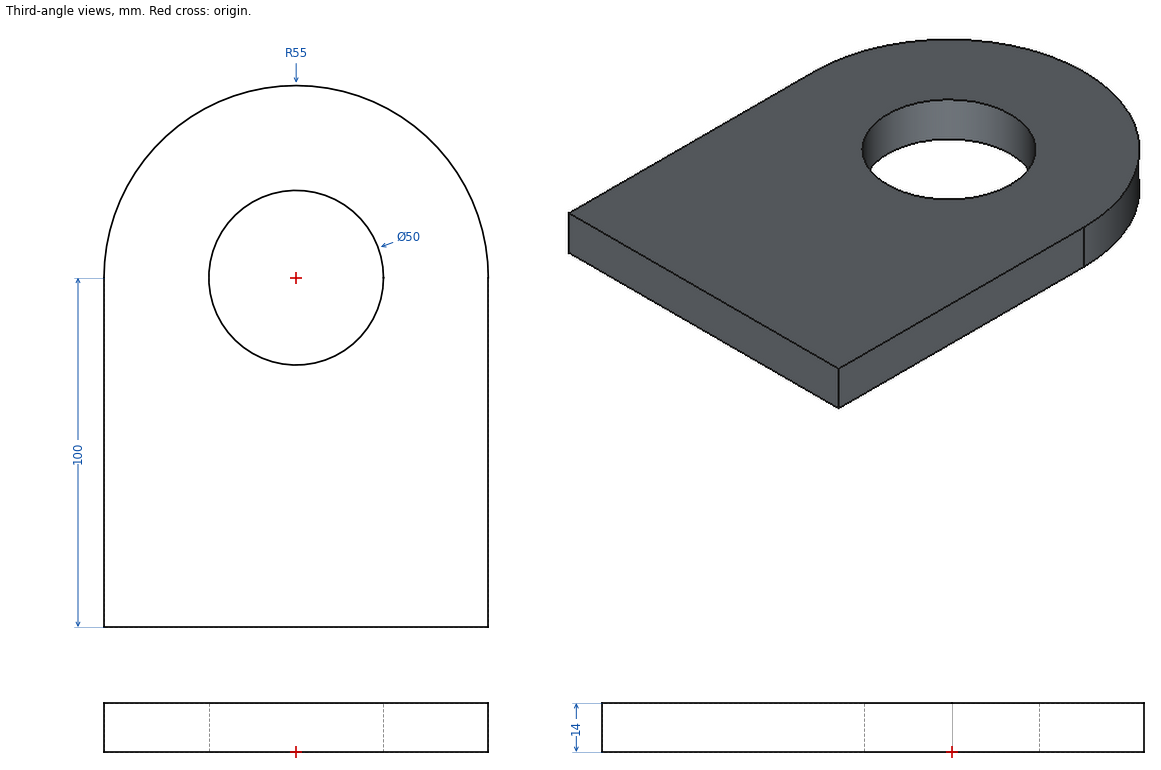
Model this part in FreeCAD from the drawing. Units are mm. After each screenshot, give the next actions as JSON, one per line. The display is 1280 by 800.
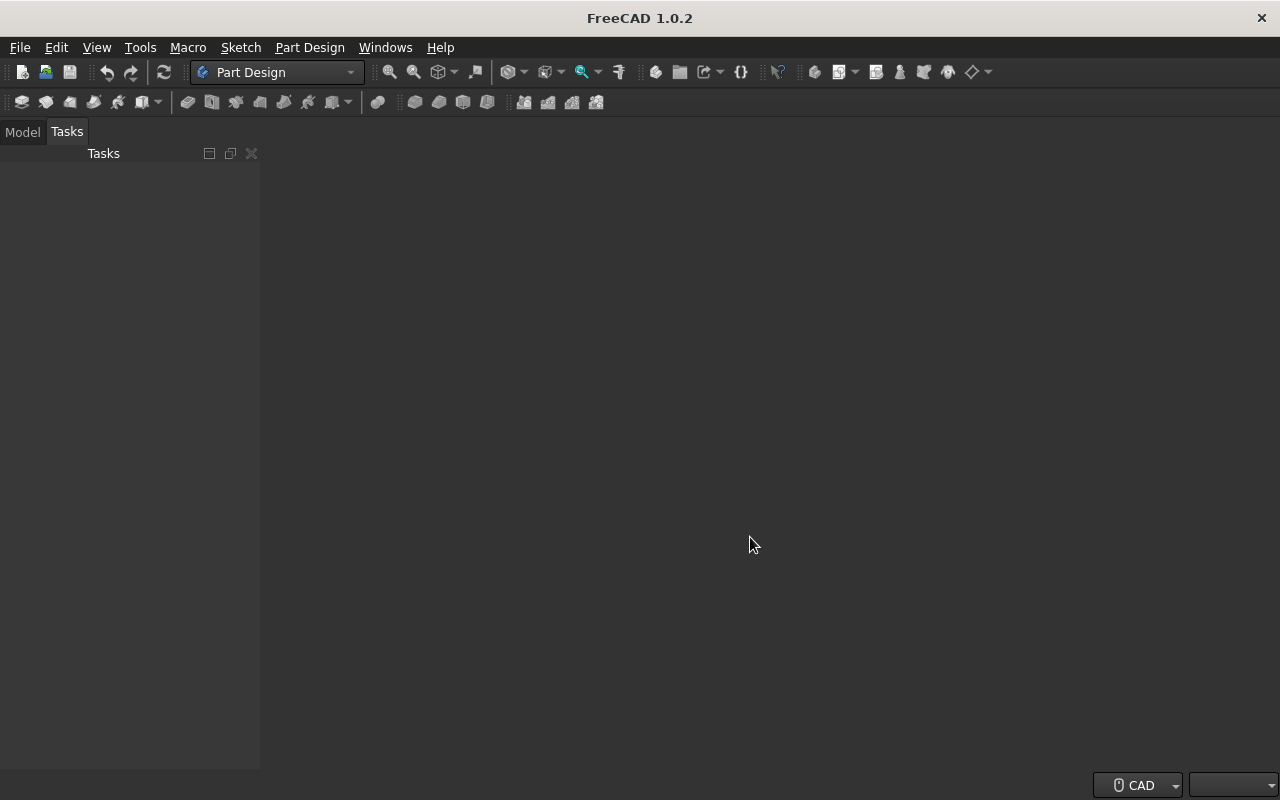
{"action": "left_click", "coordinate": [22, 72]}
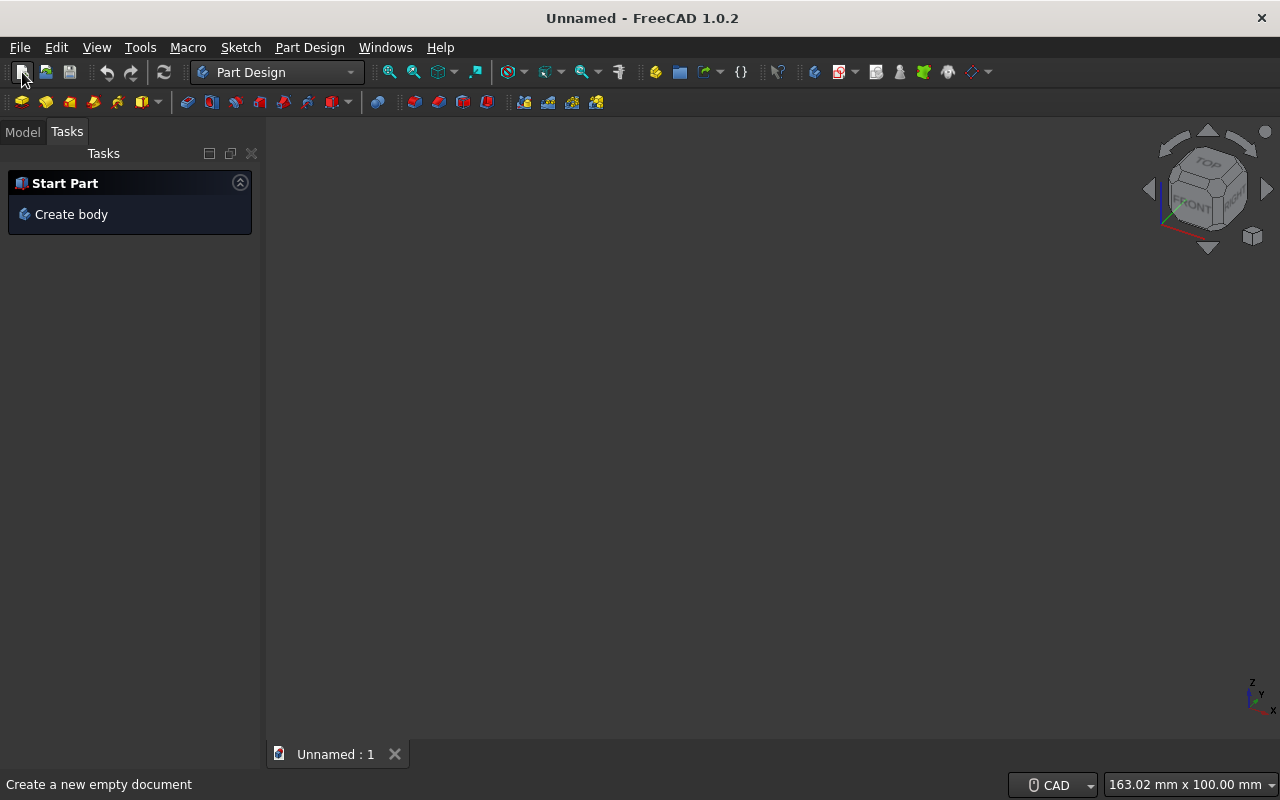
{"action": "left_click", "coordinate": [840, 72]}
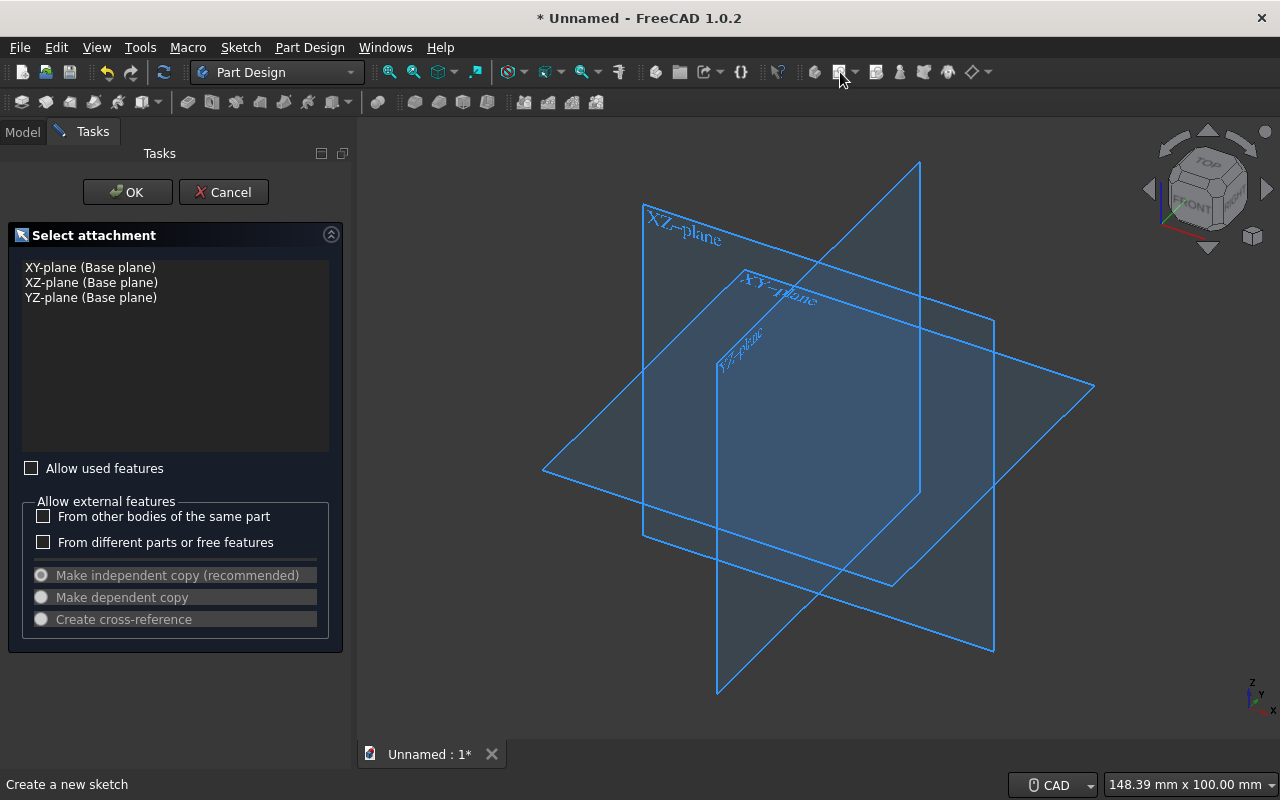
{"action": "left_click", "coordinate": [82, 268]}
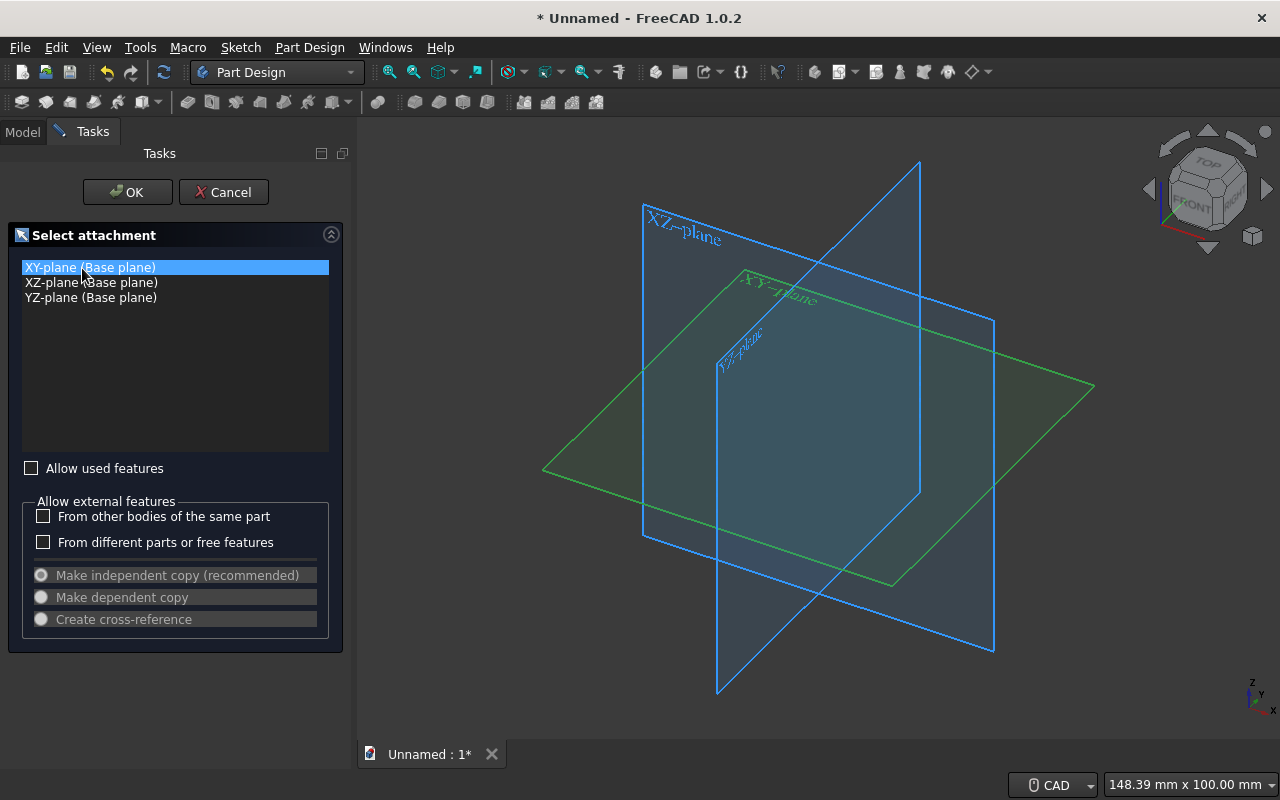
{"action": "left_click", "coordinate": [128, 192]}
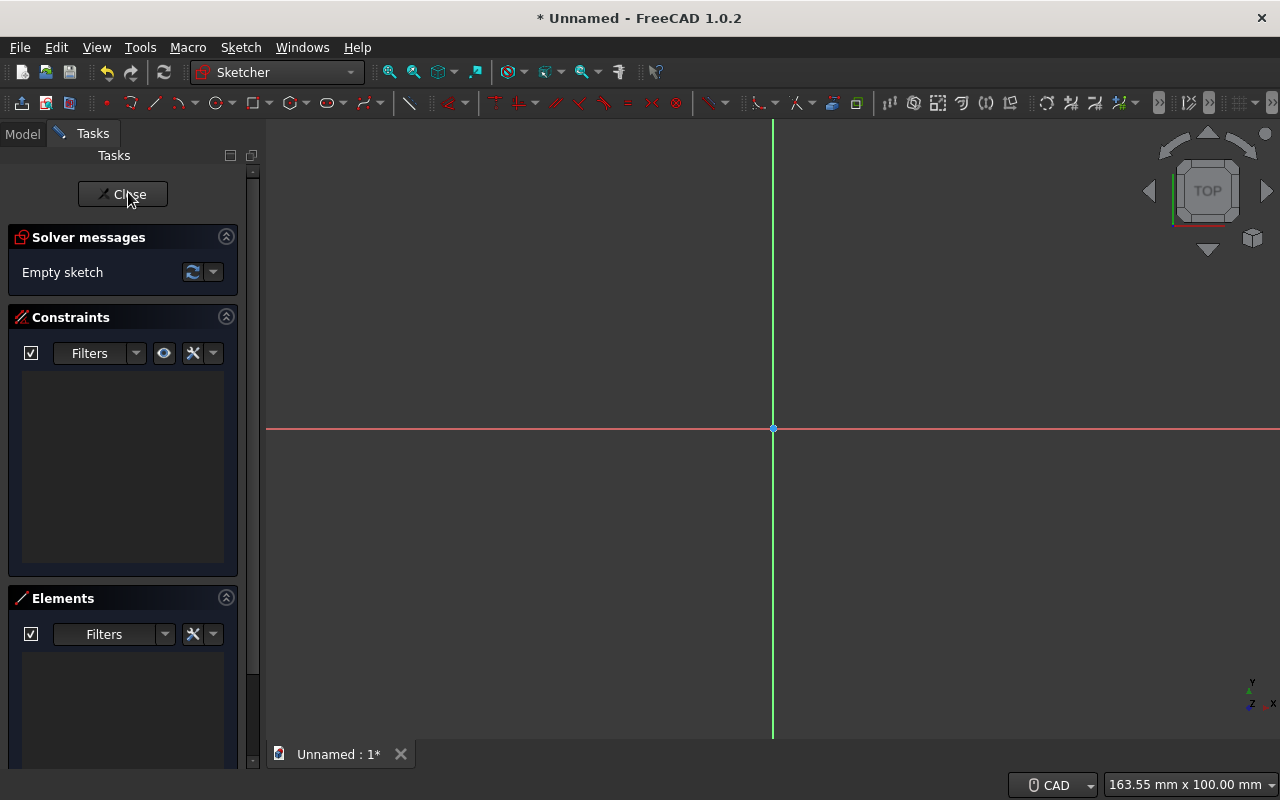
{"action": "scroll", "coordinate": [649, 315], "scroll_direction": "down", "scroll_amount": 4}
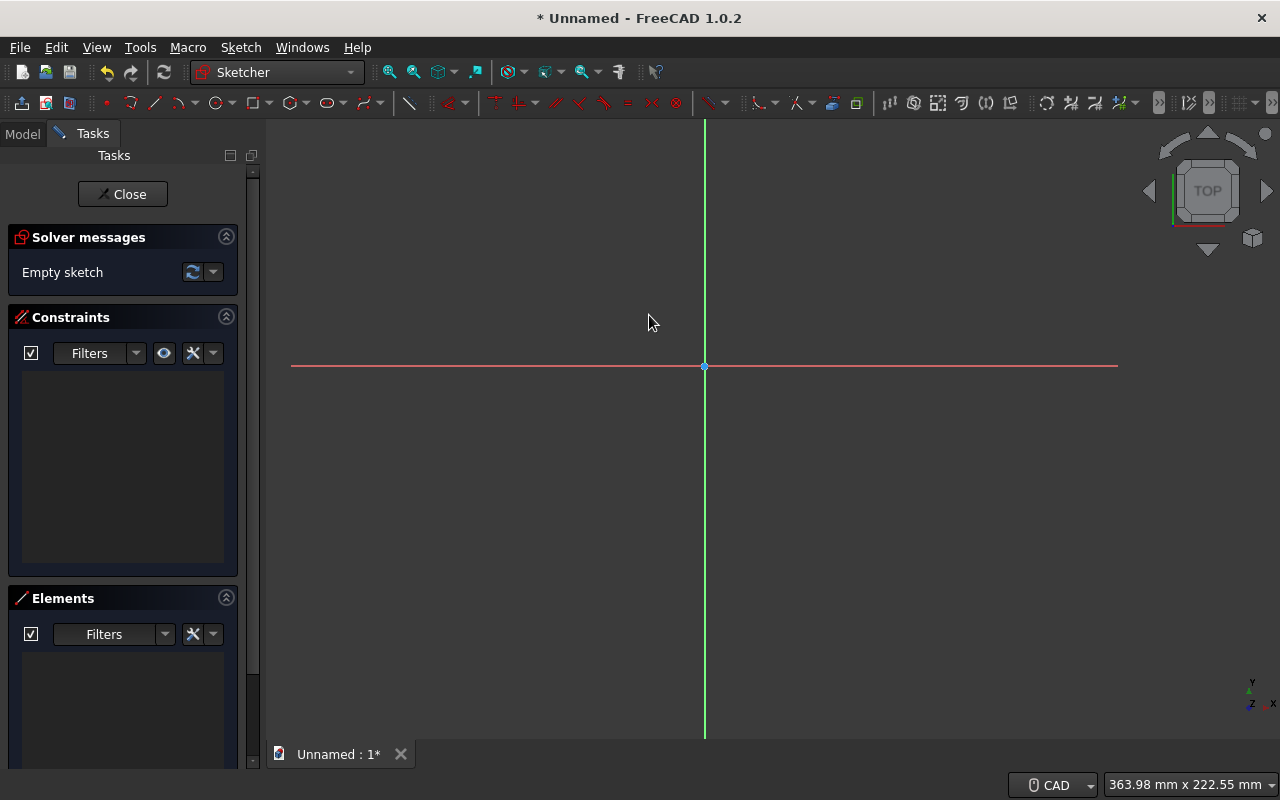
{"action": "key", "text": "g m"}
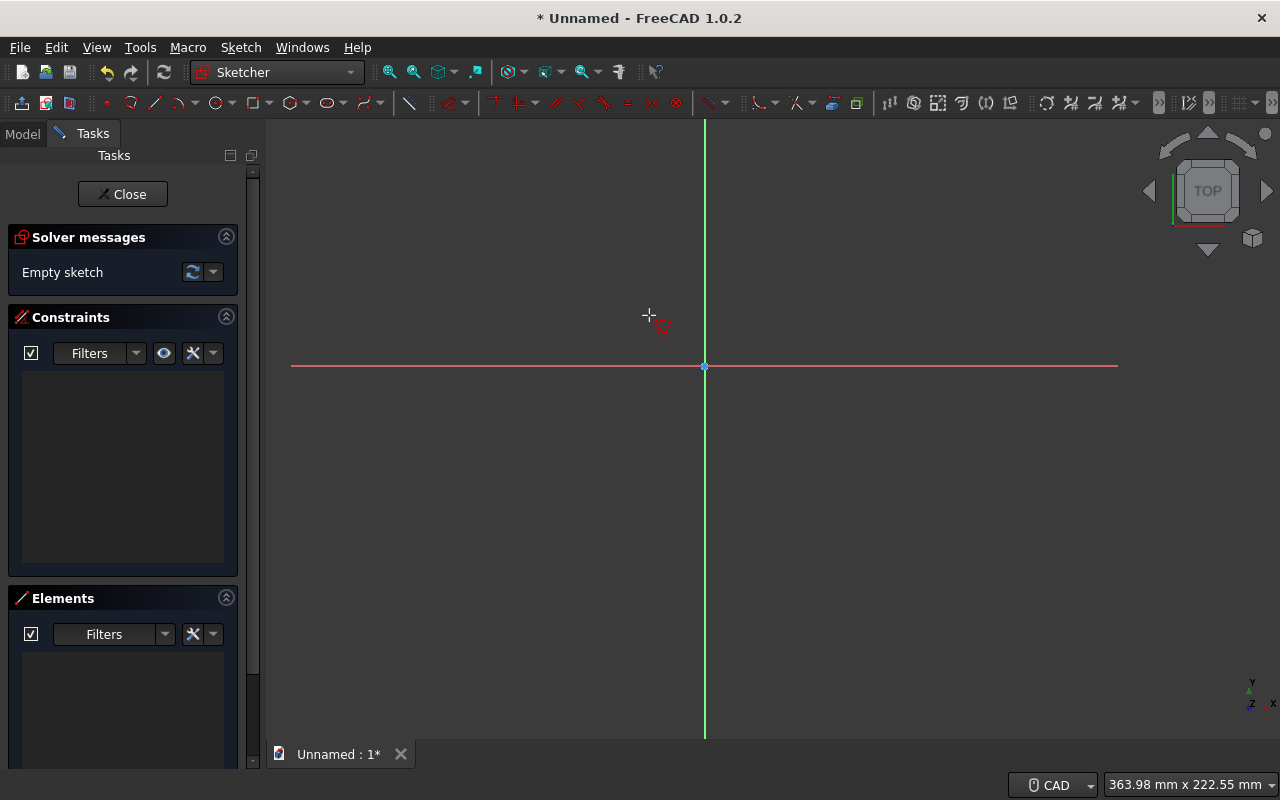
{"action": "left_click", "coordinate": [552, 366]}
{"action": "left_click", "coordinate": [552, 645]}
{"action": "left_click", "coordinate": [858, 645]}
{"action": "left_click", "coordinate": [858, 366]}
{"action": "right_click", "coordinate": [858, 366]}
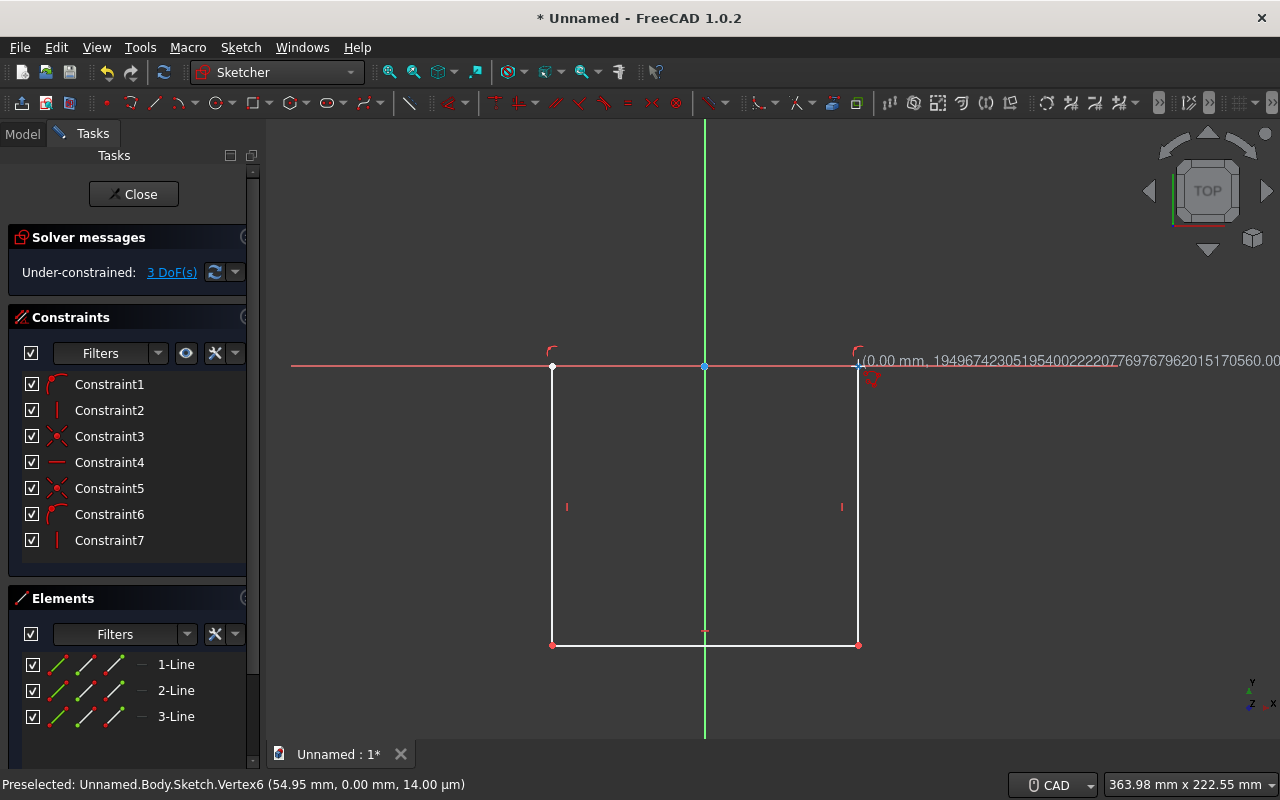
{"action": "key", "text": "g 3 a"}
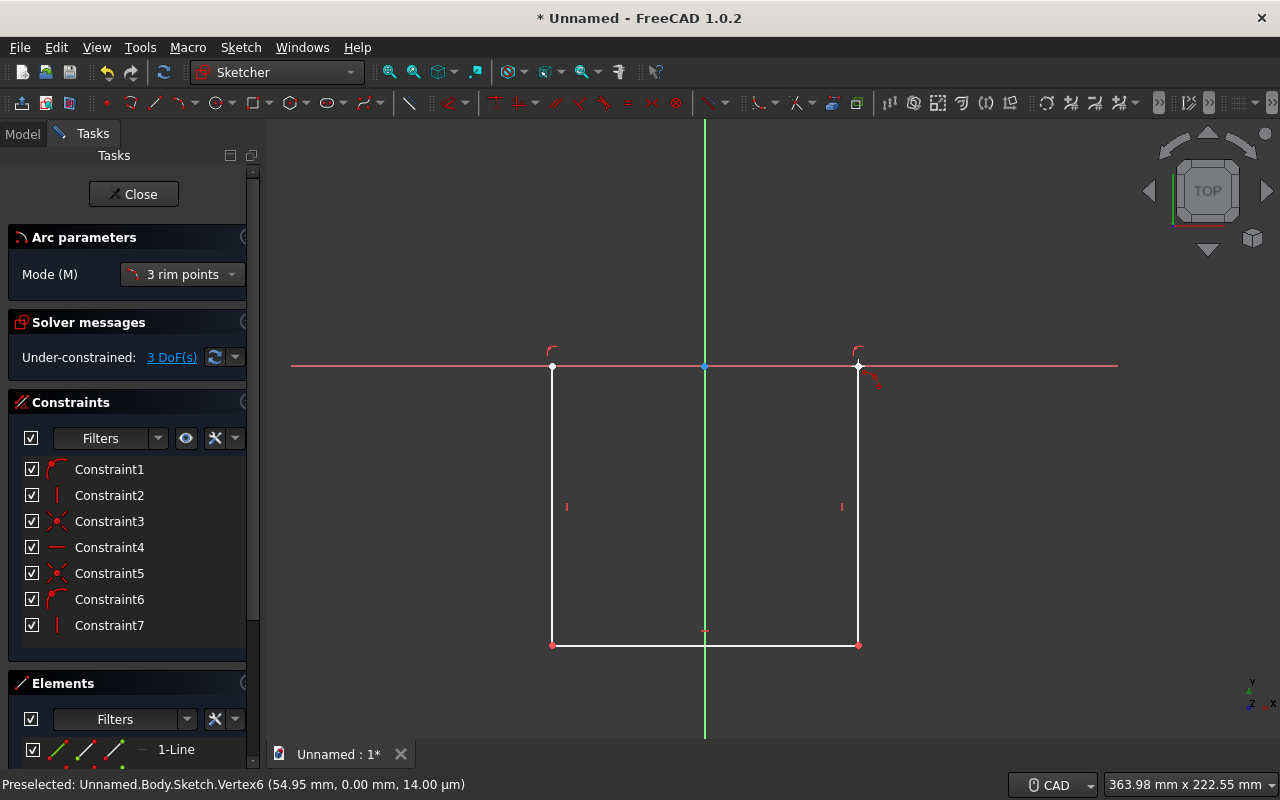
{"action": "left_click", "coordinate": [858, 366]}
{"action": "left_click", "coordinate": [552, 366]}
{"action": "left_click", "coordinate": [752, 221]}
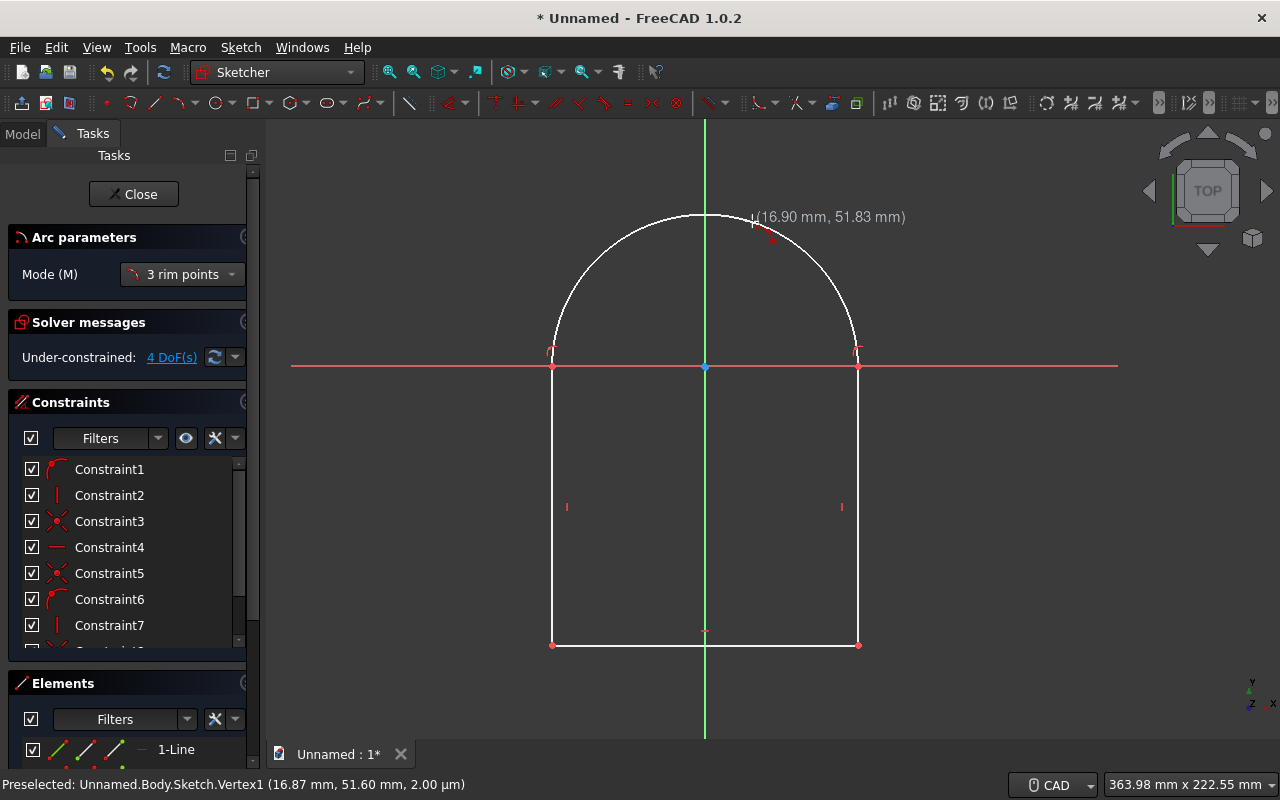
{"action": "key", "text": "g c"}